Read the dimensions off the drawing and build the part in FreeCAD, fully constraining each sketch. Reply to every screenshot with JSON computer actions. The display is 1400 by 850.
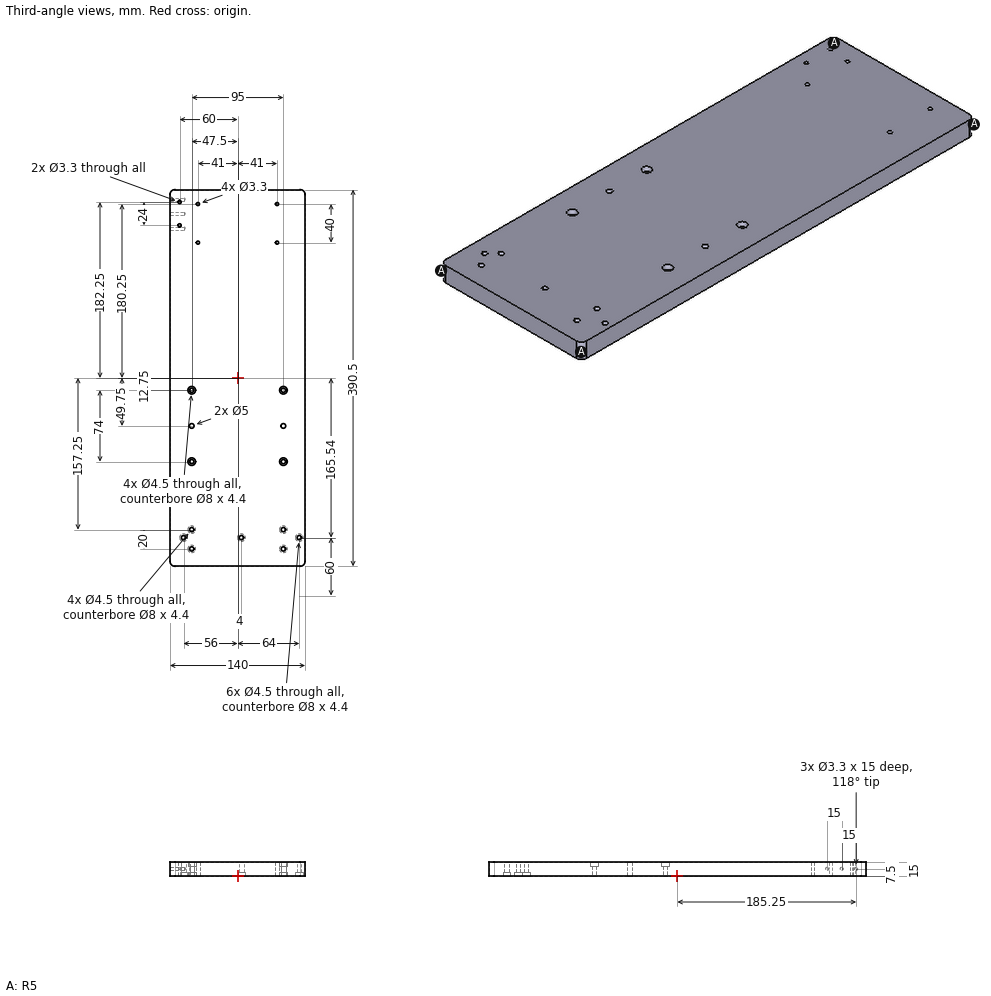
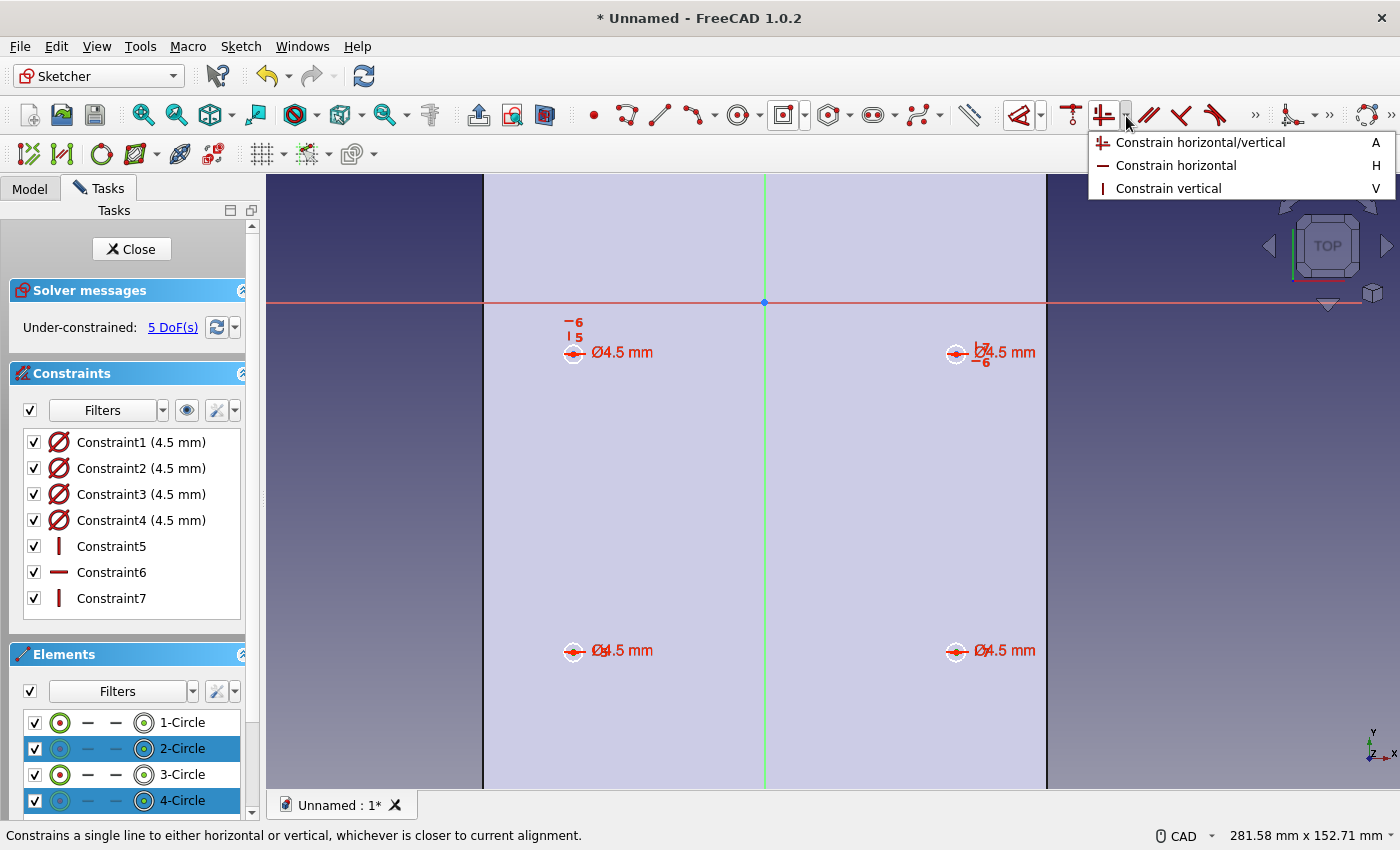
{"action": "left_click", "coordinate": [1242, 166]}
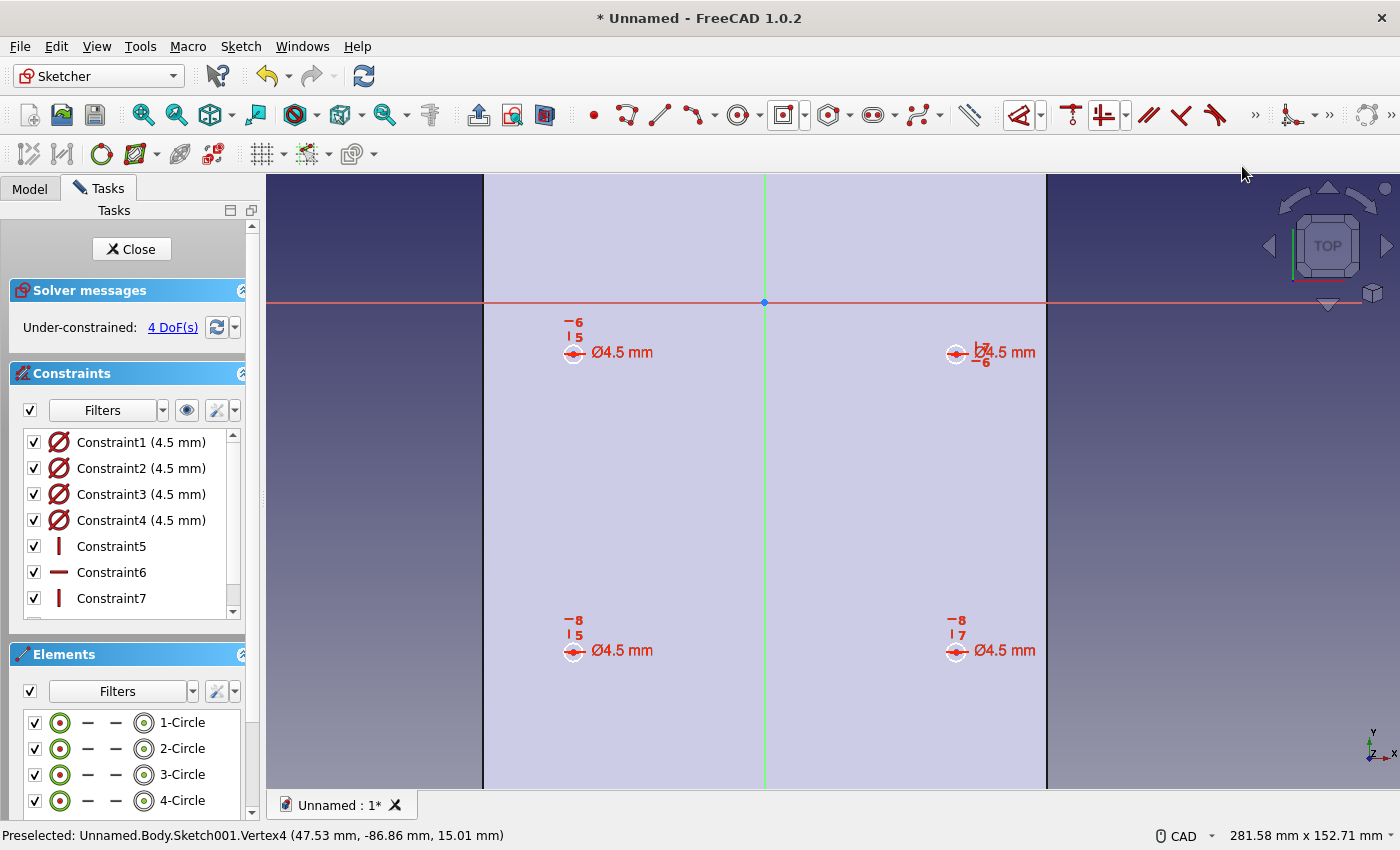
{"action": "left_click", "coordinate": [1018, 116]}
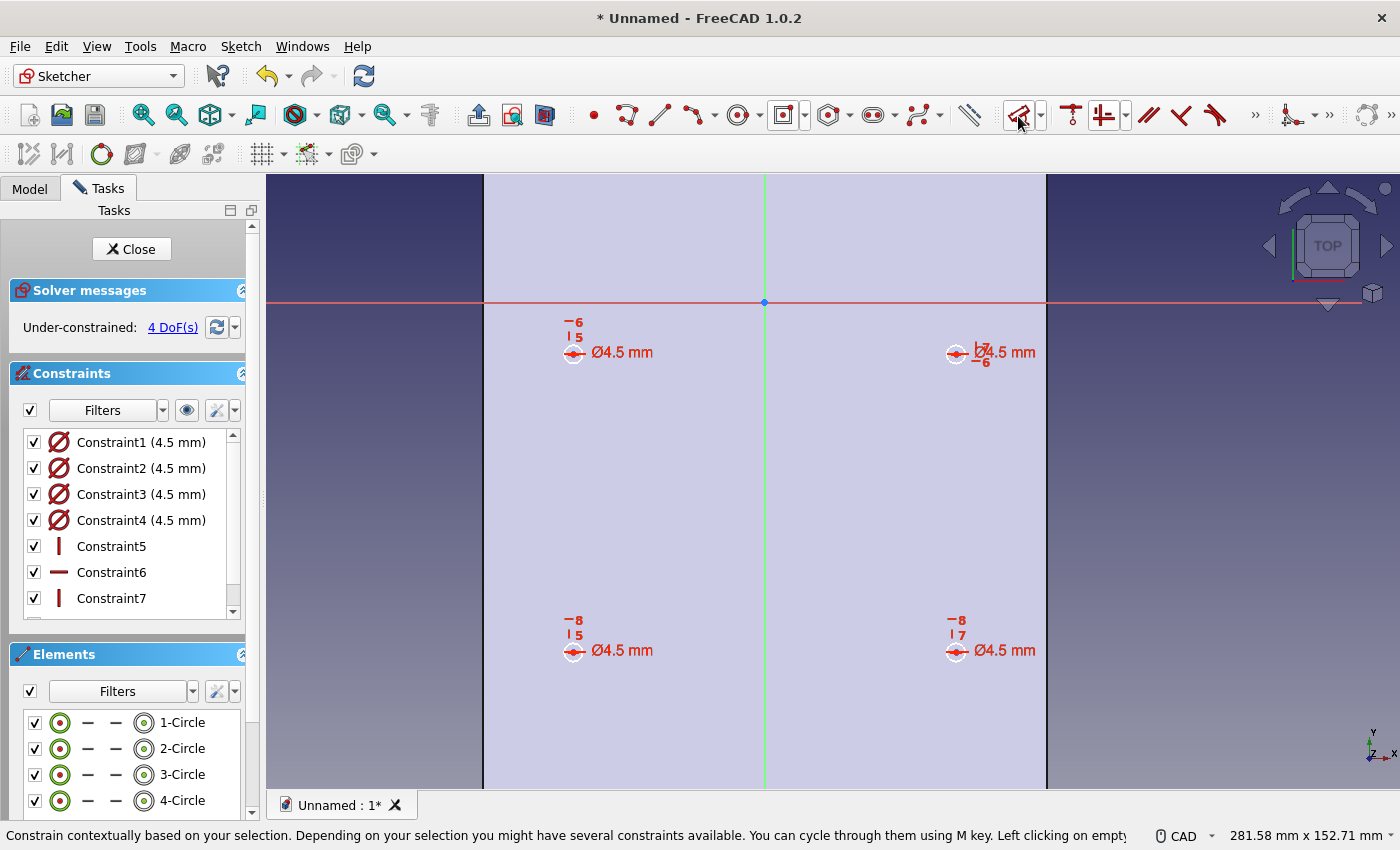
{"action": "left_click", "coordinate": [573, 354]}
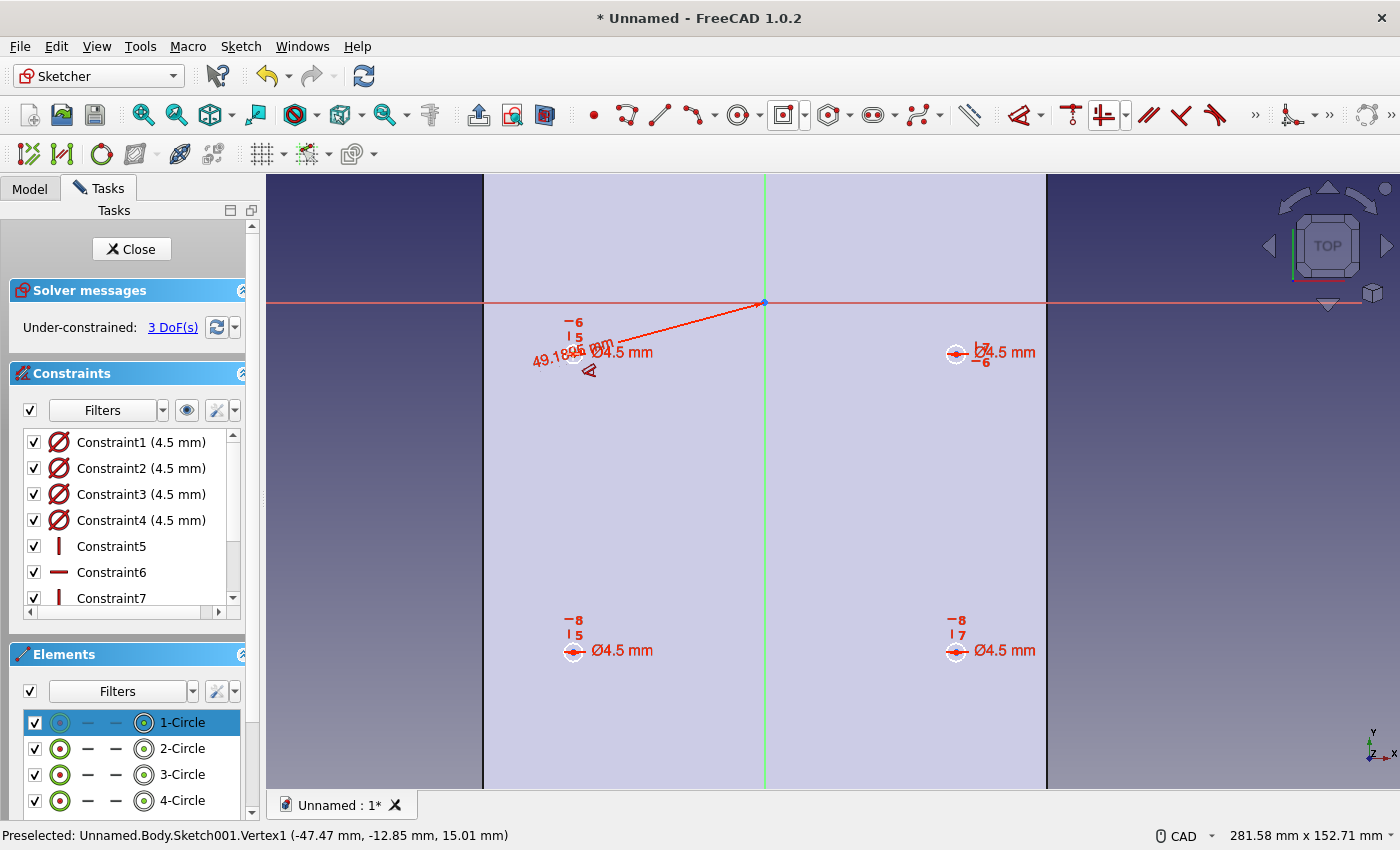
{"action": "left_click", "coordinate": [573, 652]}
{"action": "left_click", "coordinate": [539, 503]}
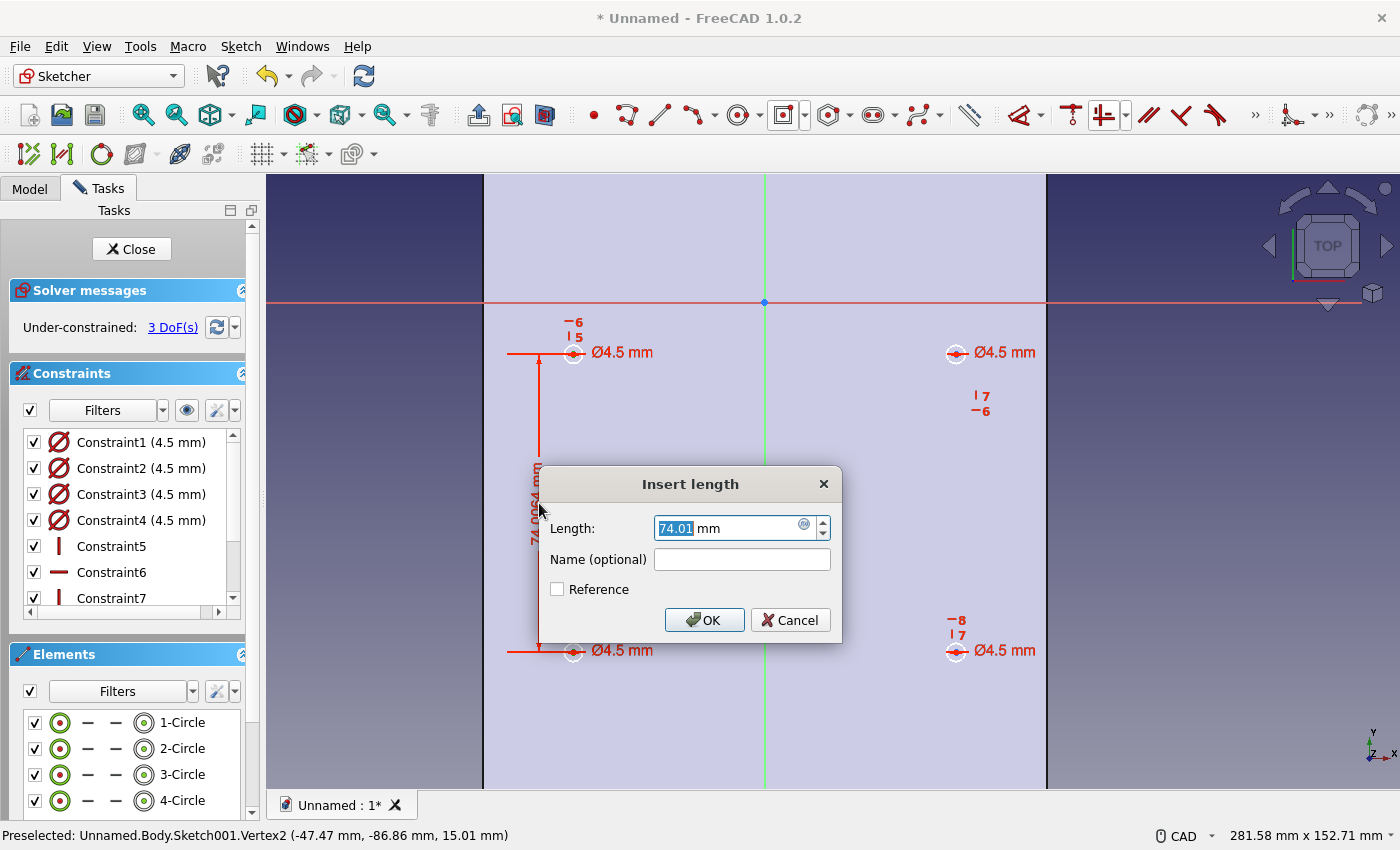
{"action": "type", "text": "74"}
{"action": "key", "text": "Return"}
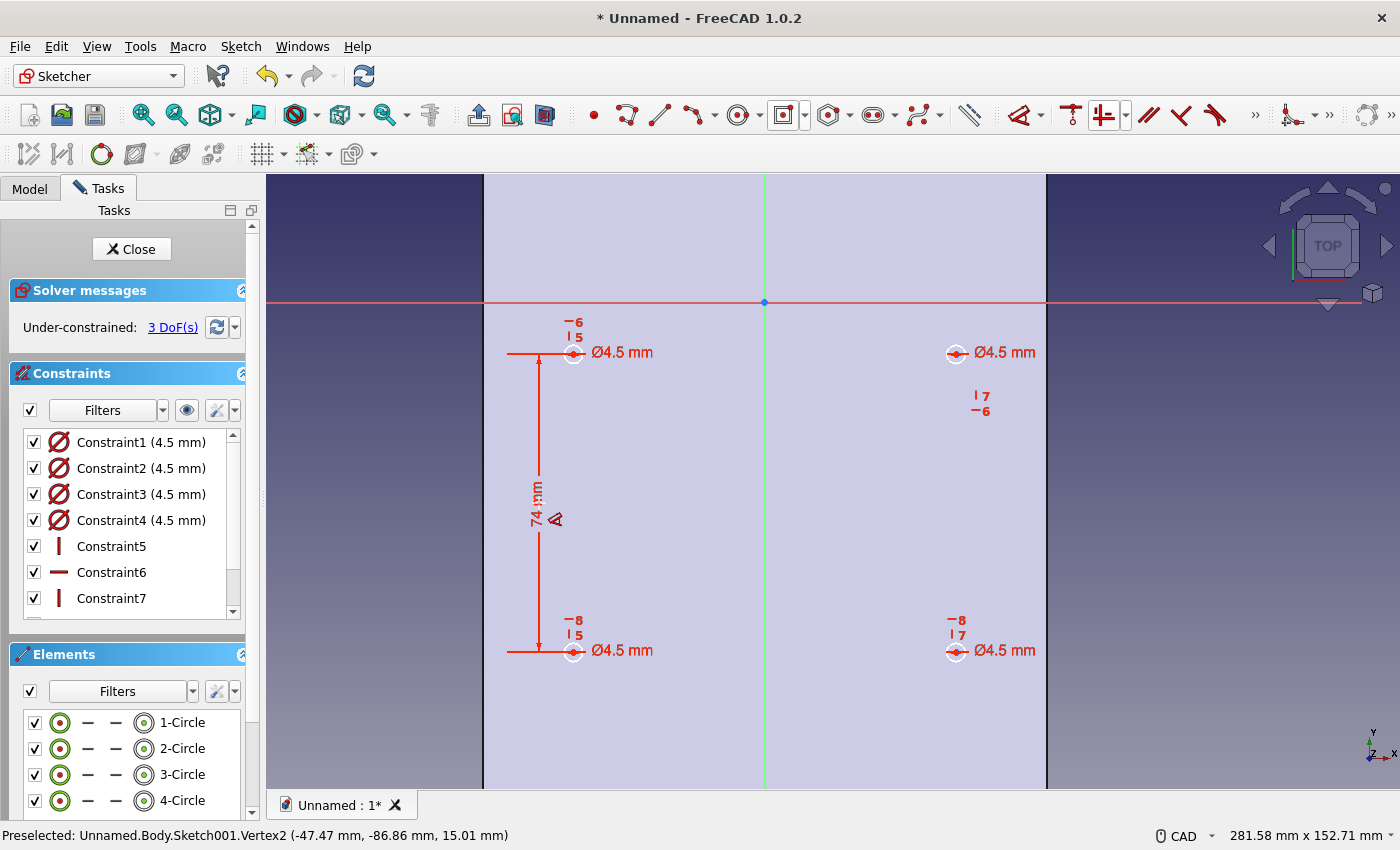
{"action": "left_click", "coordinate": [573, 354]}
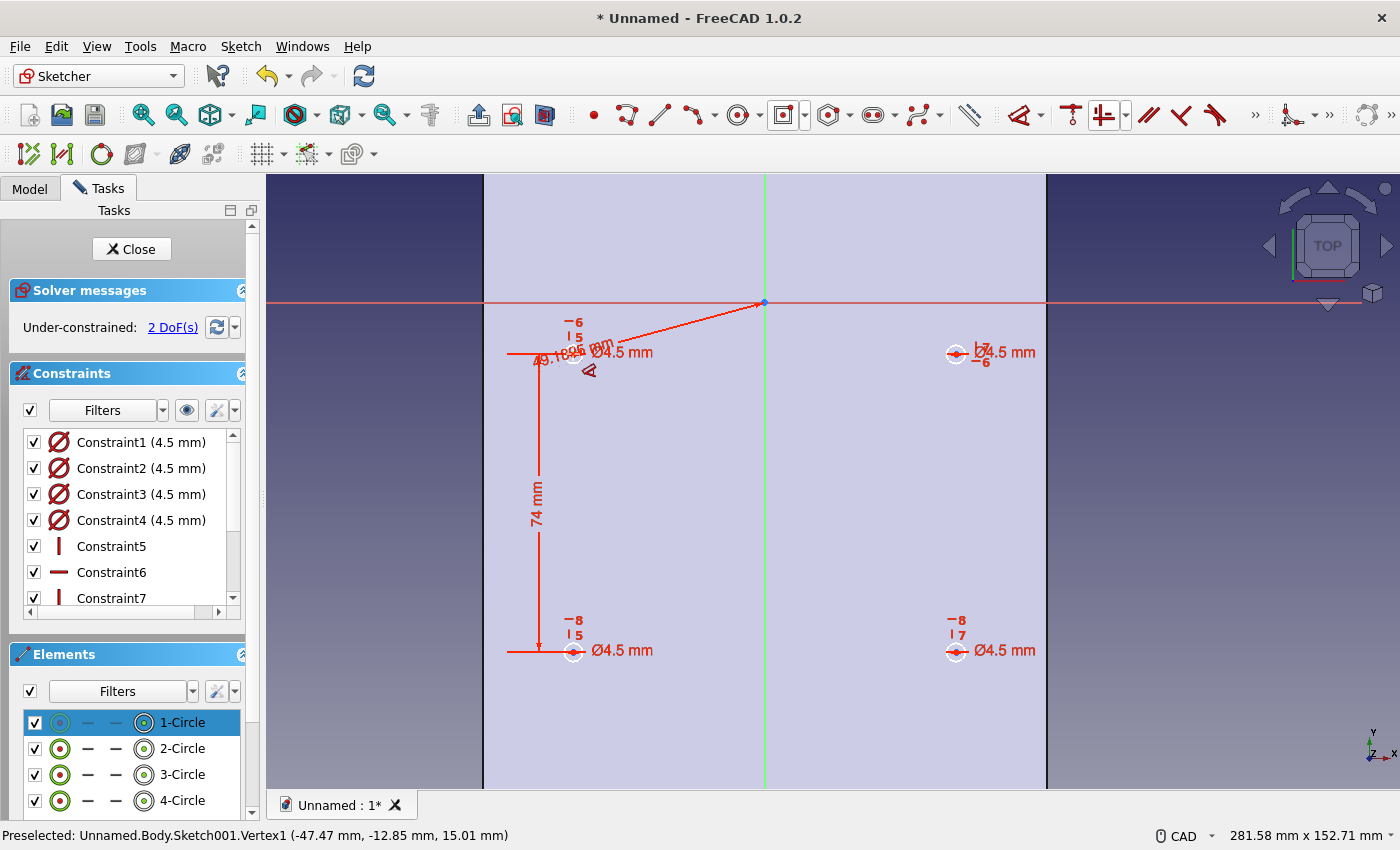
{"action": "left_click", "coordinate": [956, 354]}
{"action": "left_click", "coordinate": [677, 320]}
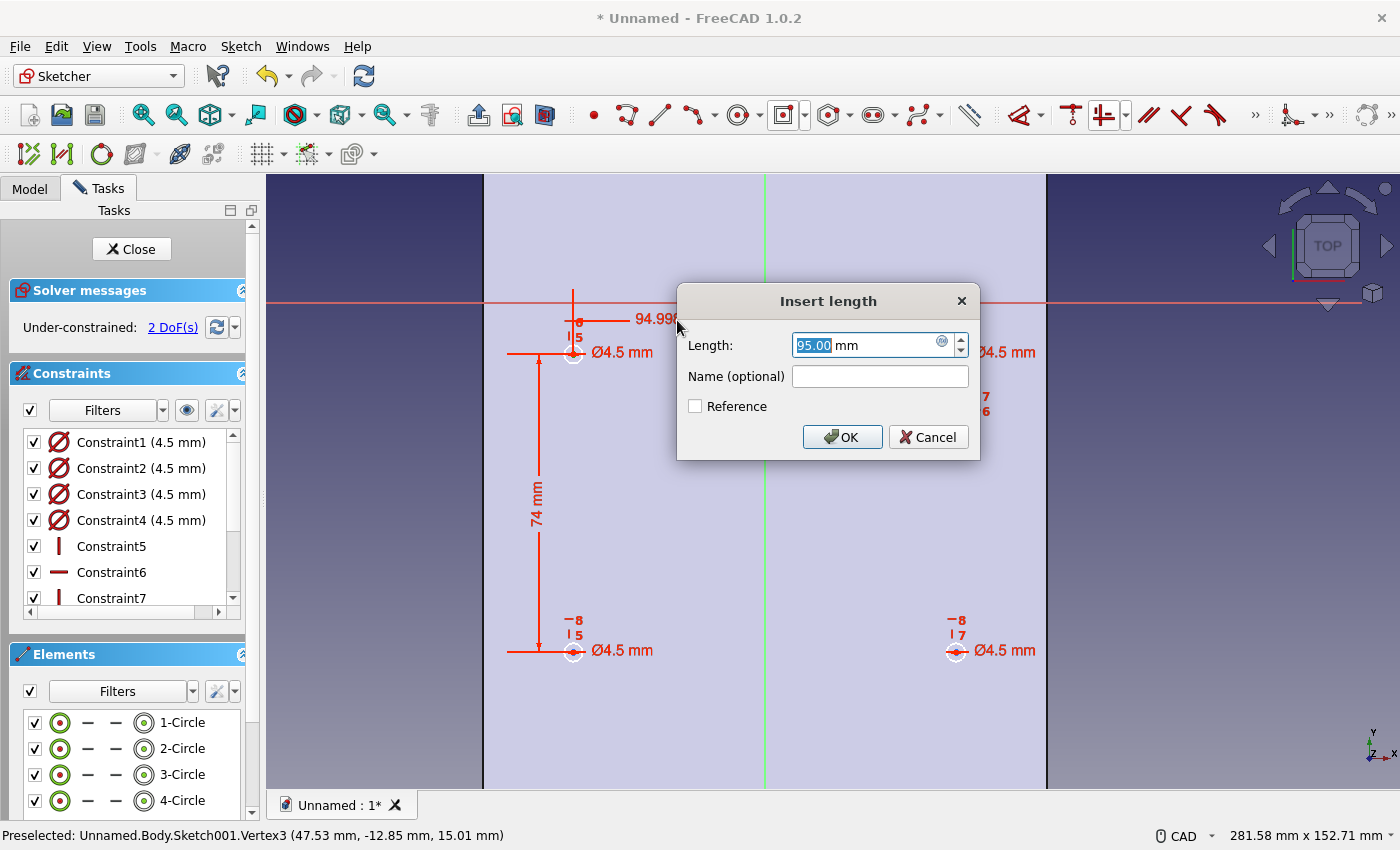
{"action": "type", "text": "95"}
{"action": "key", "text": "Return"}